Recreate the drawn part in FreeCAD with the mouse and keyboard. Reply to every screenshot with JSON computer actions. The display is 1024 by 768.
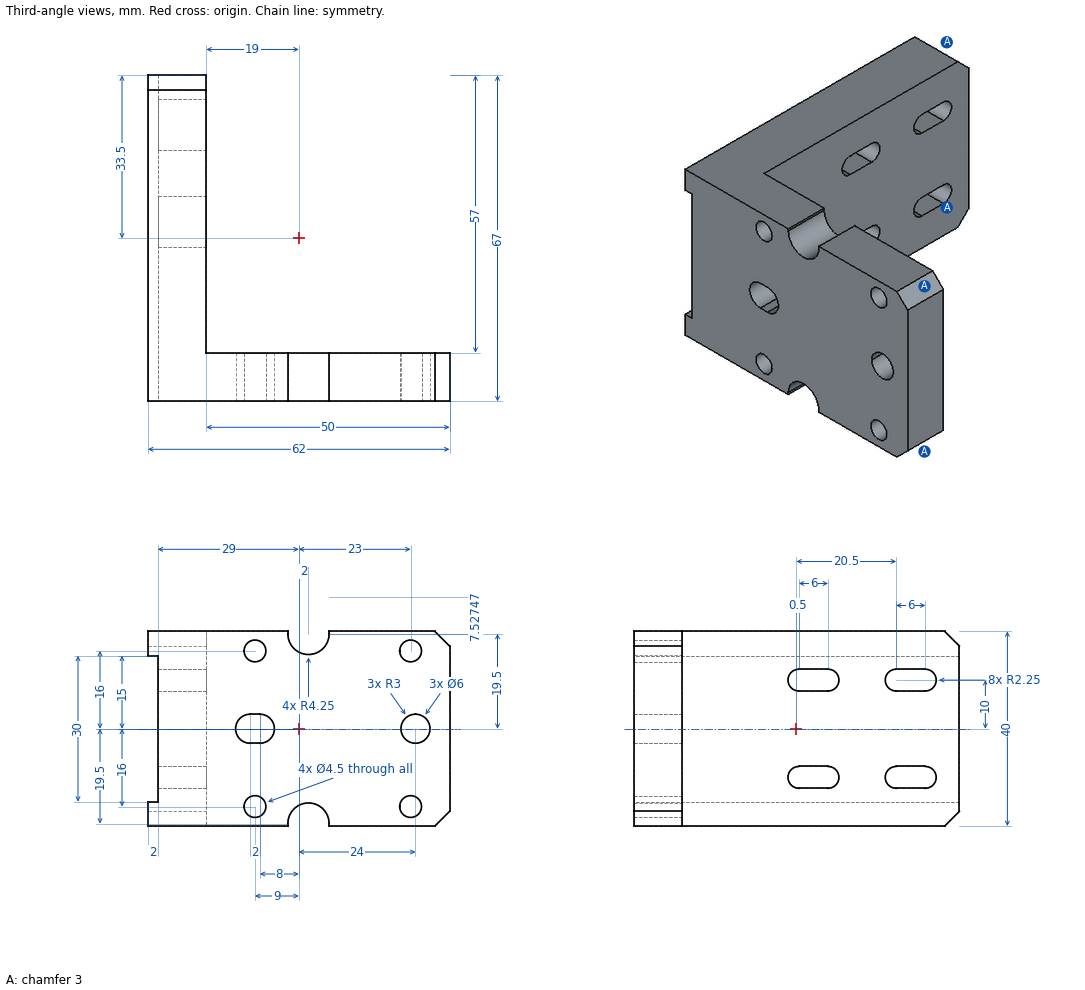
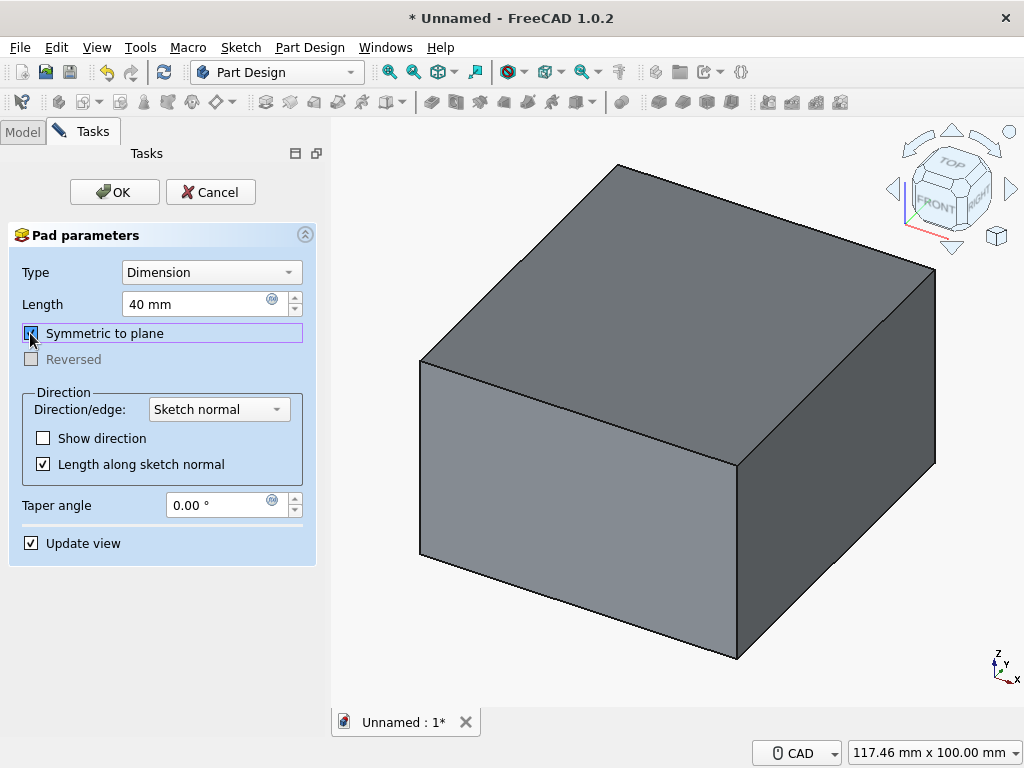
{"action": "left_click", "coordinate": [115, 192]}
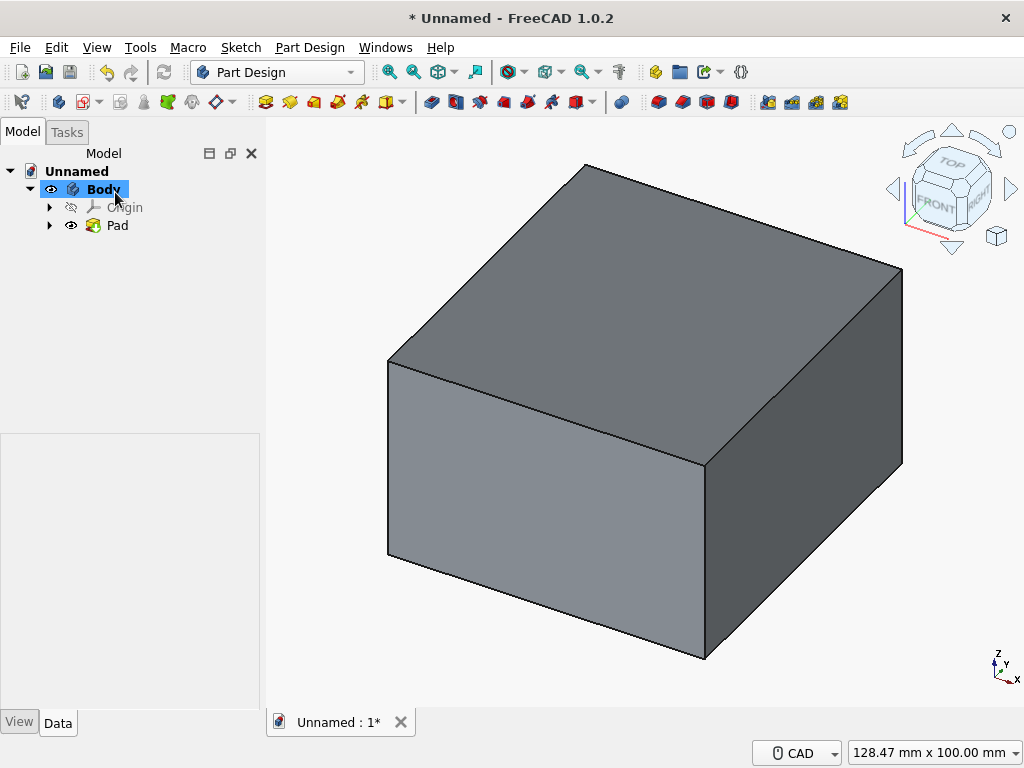
{"action": "left_click", "coordinate": [645, 314]}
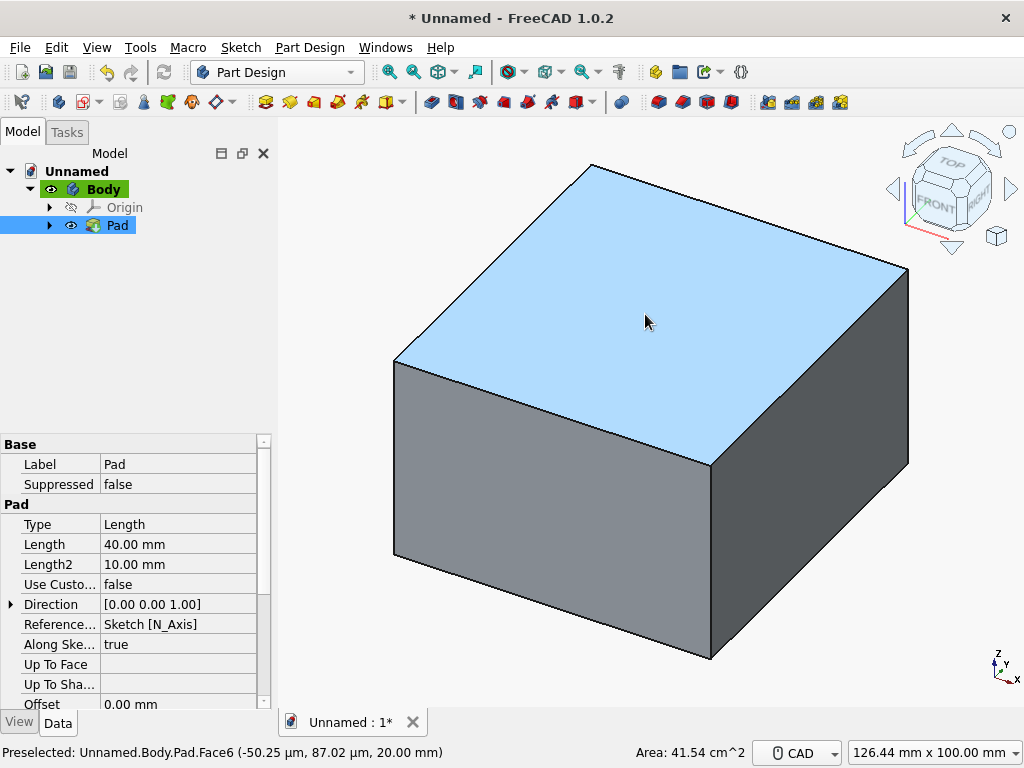
{"action": "left_click", "coordinate": [84, 102]}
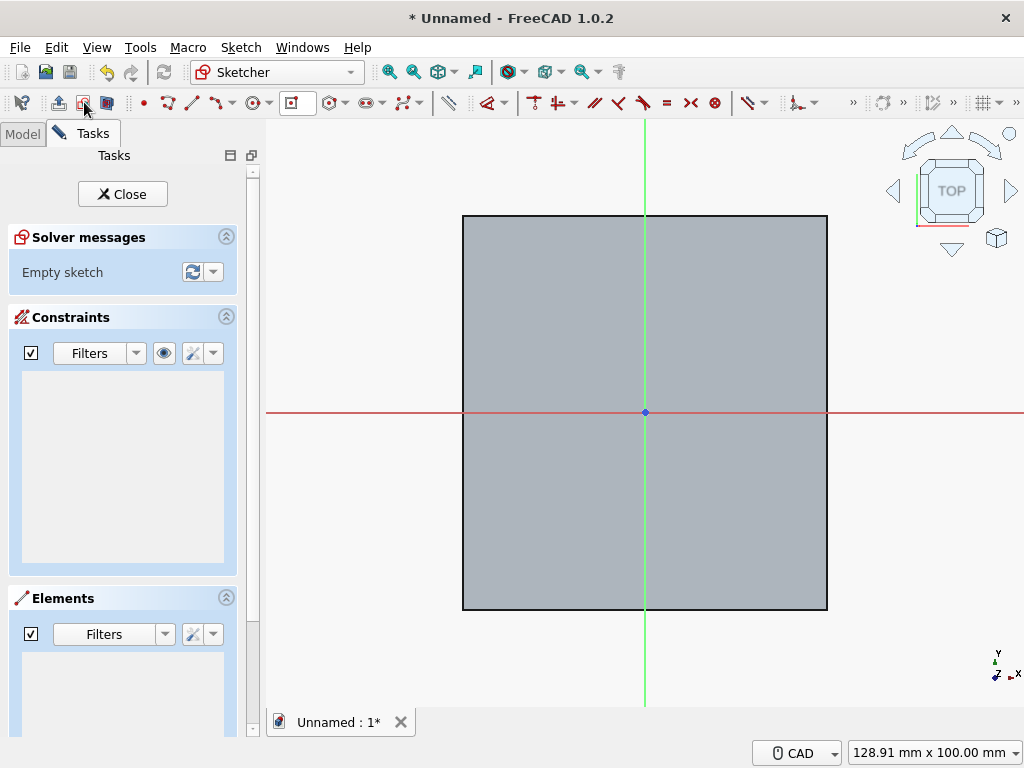
{"action": "left_click", "coordinate": [310, 104]}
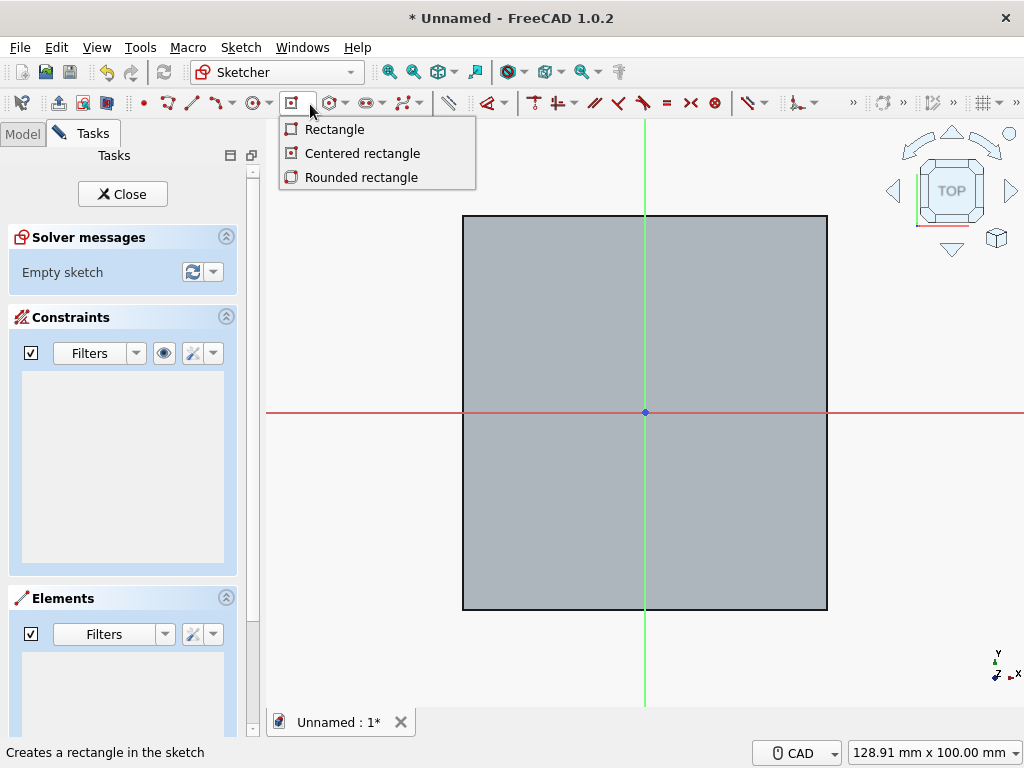
{"action": "left_click", "coordinate": [378, 129]}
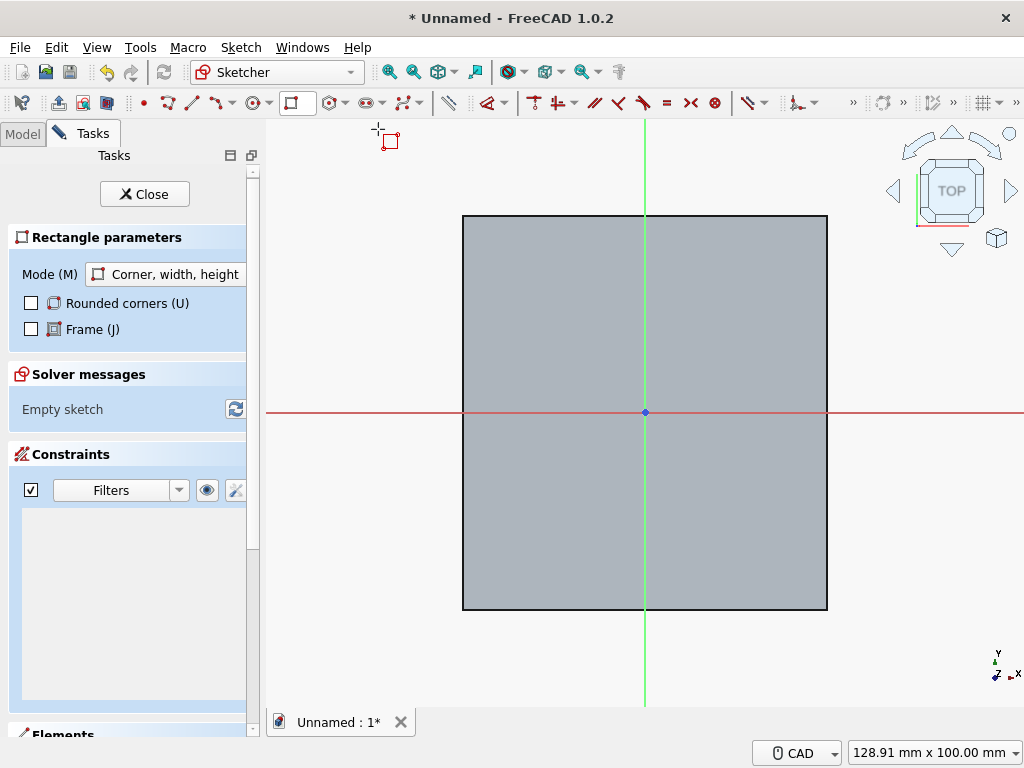
{"action": "left_click", "coordinate": [533, 216]}
{"action": "mouse_move", "coordinate": [827, 551]}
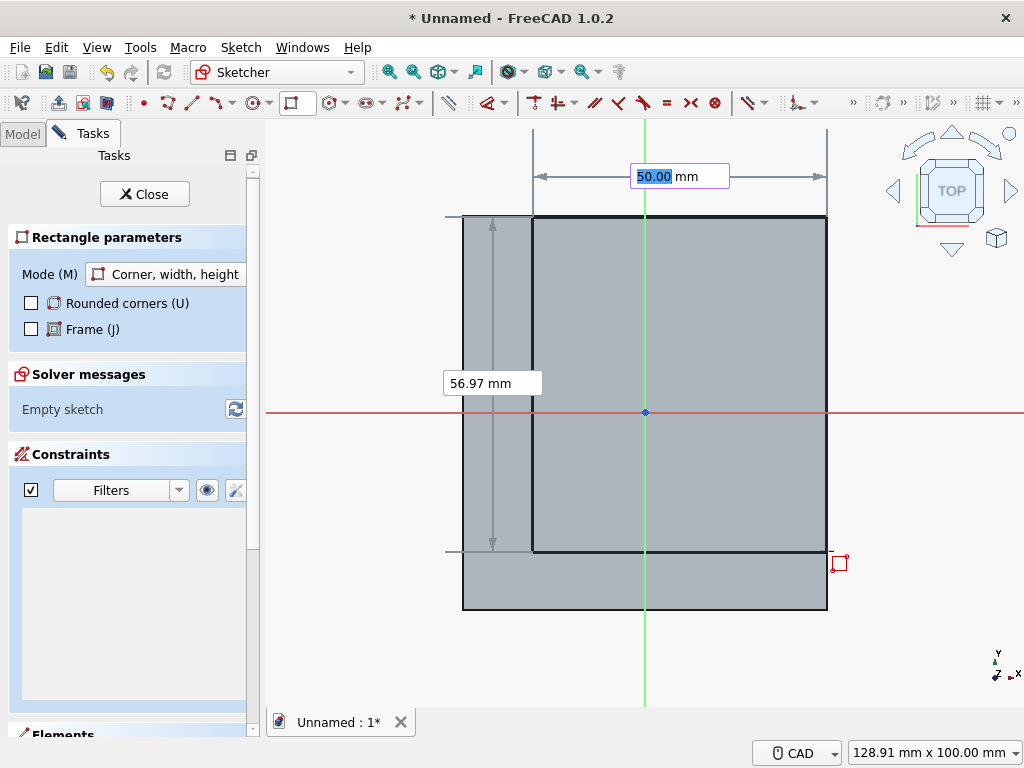
{"action": "type", "text": "50"}
{"action": "key", "text": "Tab"}
{"action": "type", "text": "57"}
{"action": "key", "text": "Return"}
{"action": "key", "text": "Escape"}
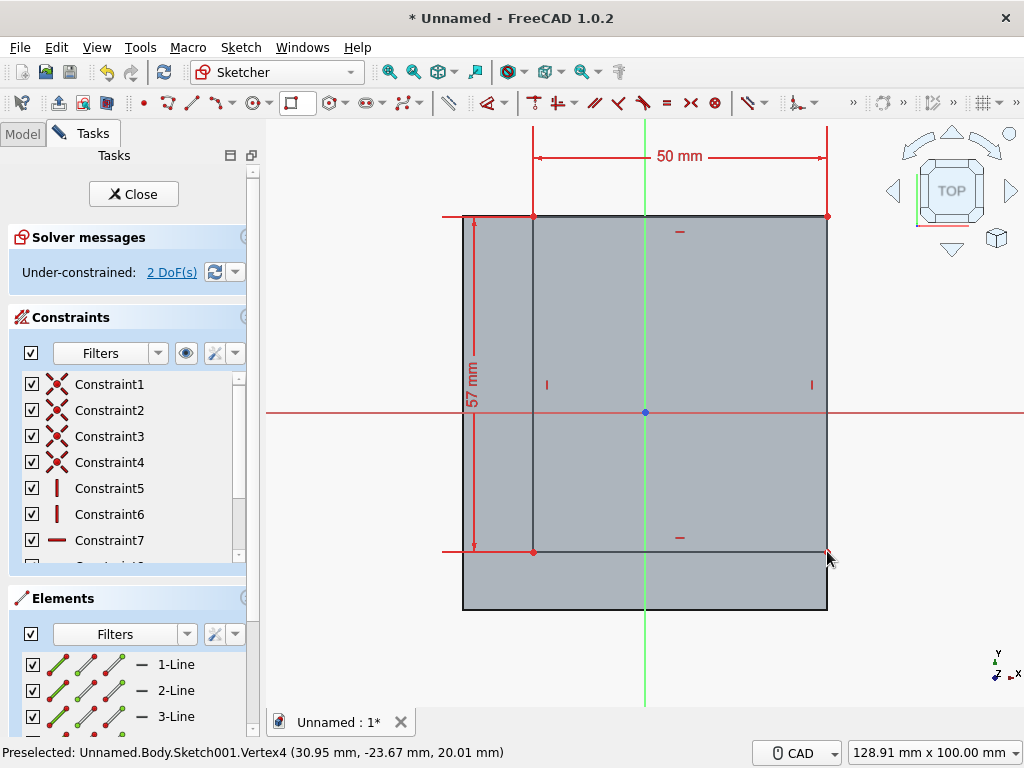
{"action": "left_click", "coordinate": [488, 104]}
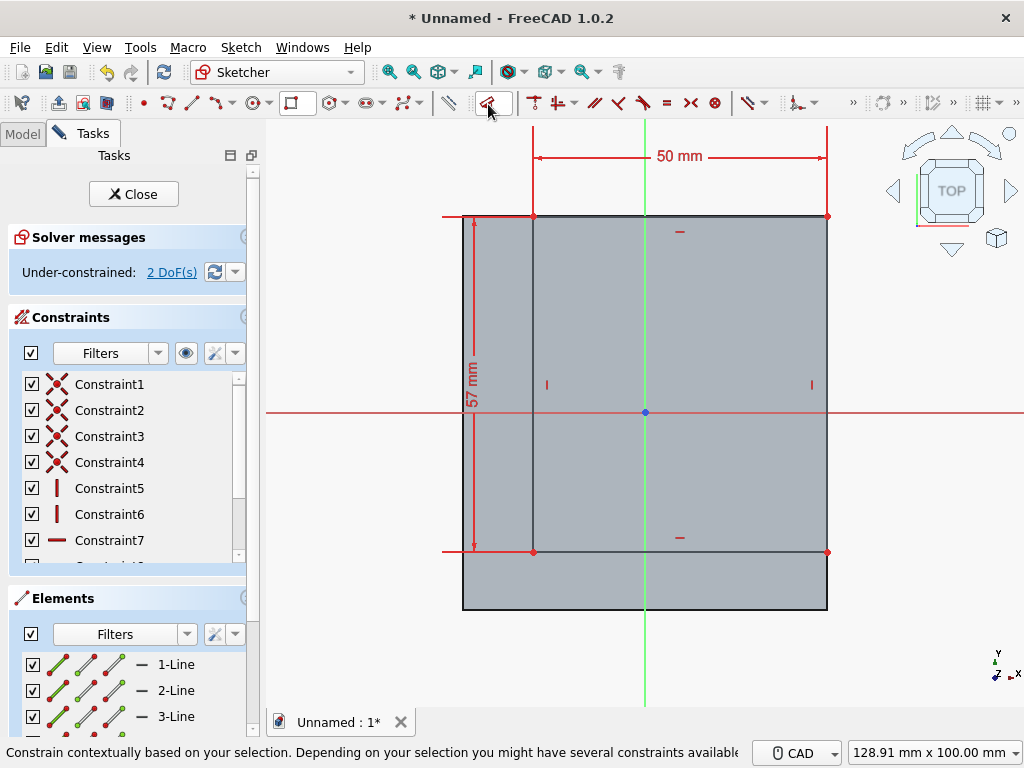
{"action": "left_click", "coordinate": [533, 217]}
{"action": "left_click", "coordinate": [589, 183]}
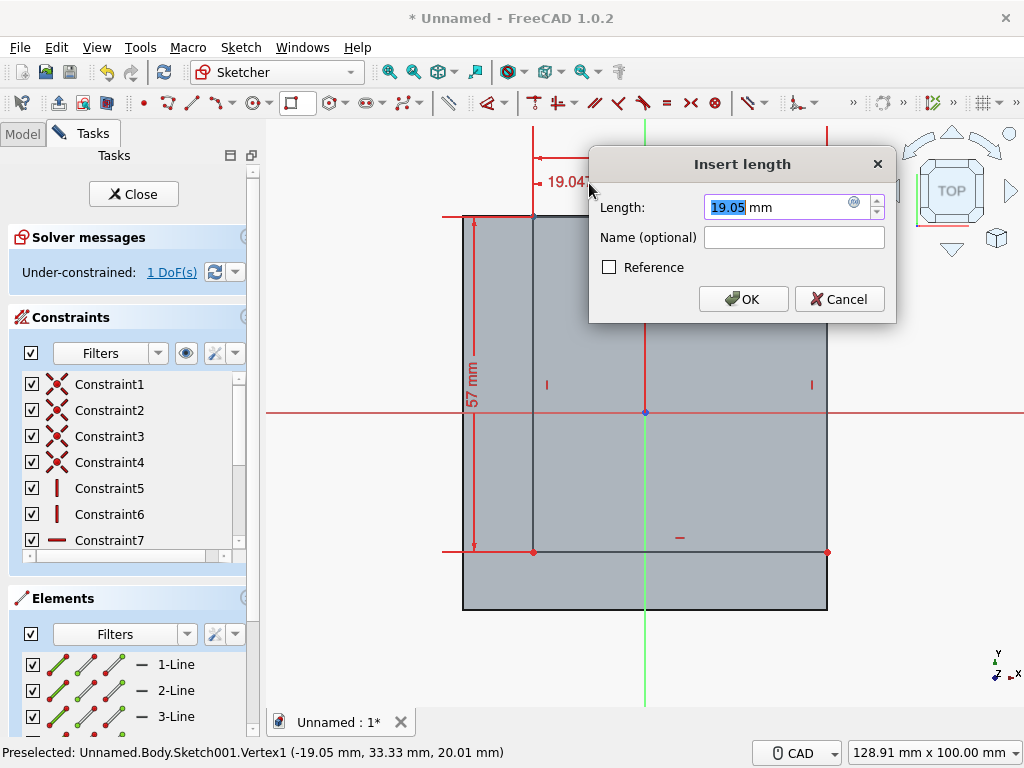
{"action": "type", "text": "19"}
{"action": "key", "text": "Return"}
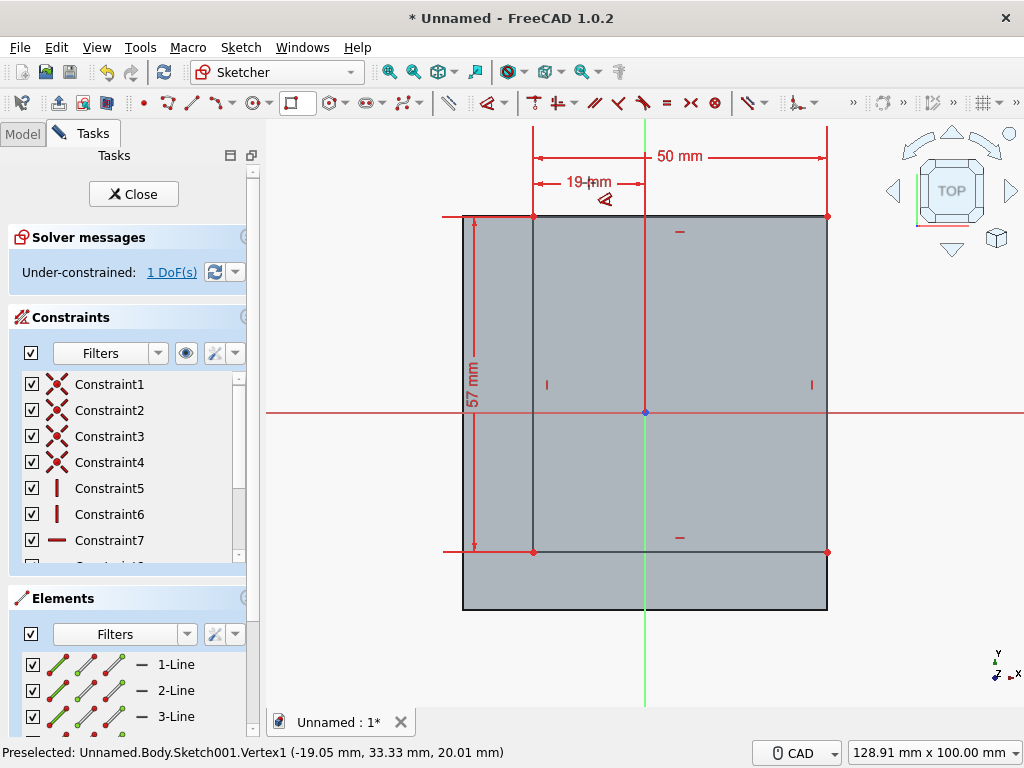
{"action": "left_click", "coordinate": [533, 217]}
{"action": "left_click", "coordinate": [499, 315]}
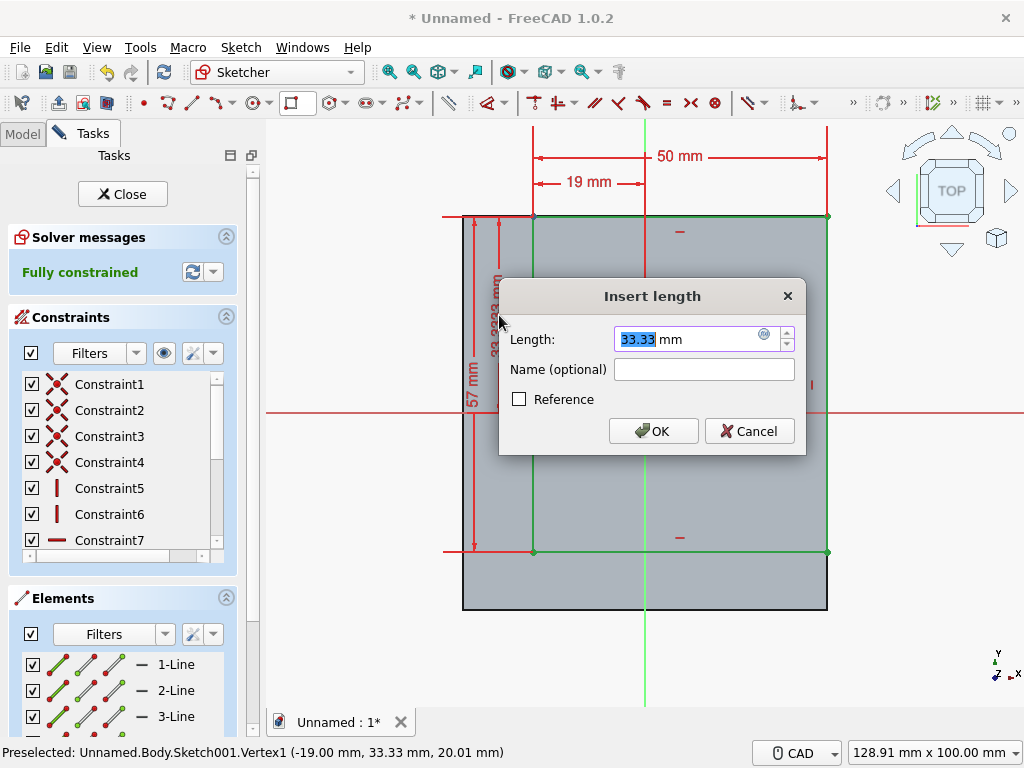
{"action": "type", "text": "33.5"}
{"action": "key", "text": "Return"}
{"action": "key", "text": "Escape"}